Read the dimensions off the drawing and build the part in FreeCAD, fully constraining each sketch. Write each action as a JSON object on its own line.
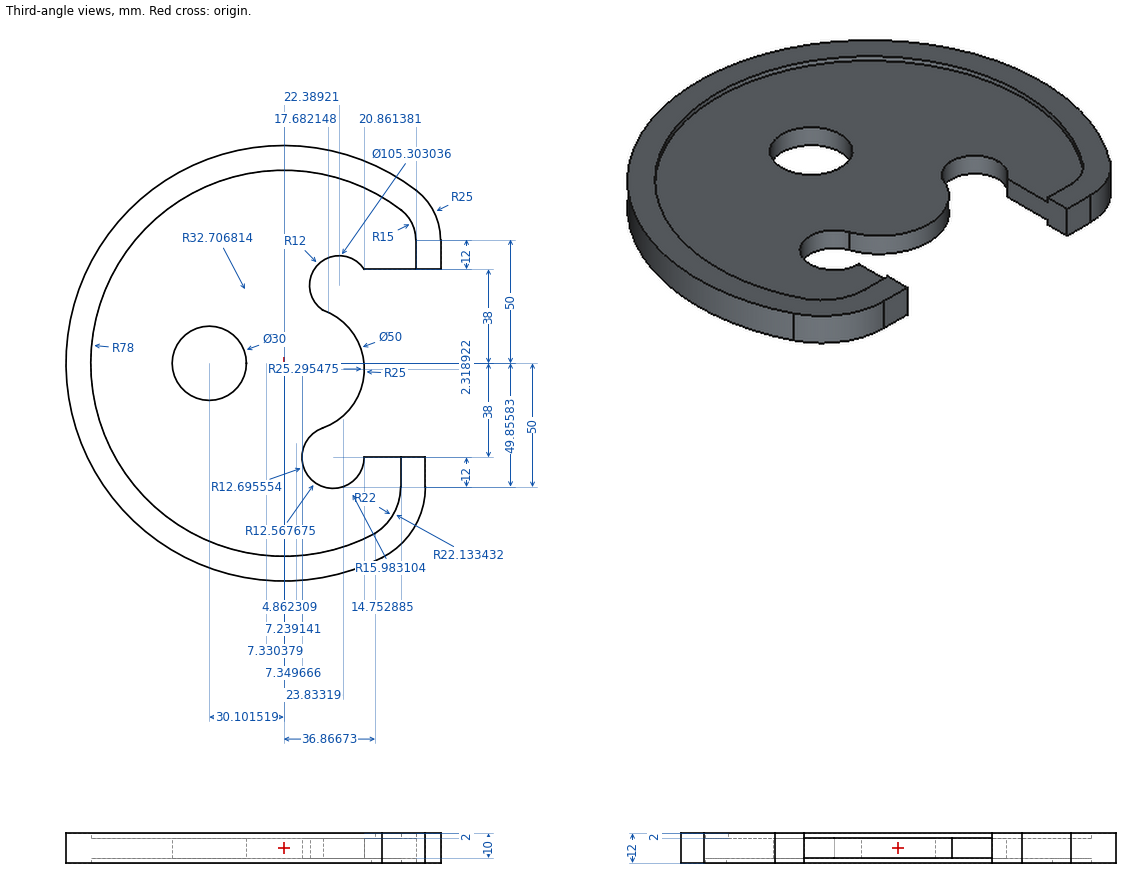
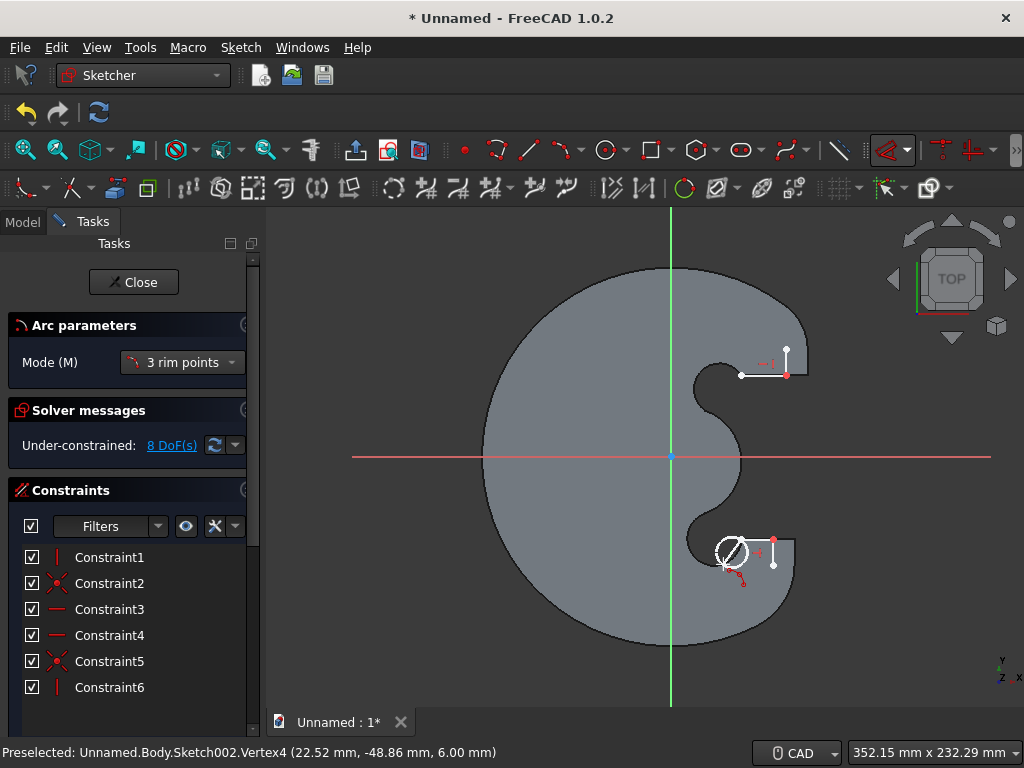
{"action": "scroll", "coordinate": [736, 554], "scroll_direction": "up", "scroll_amount": 6}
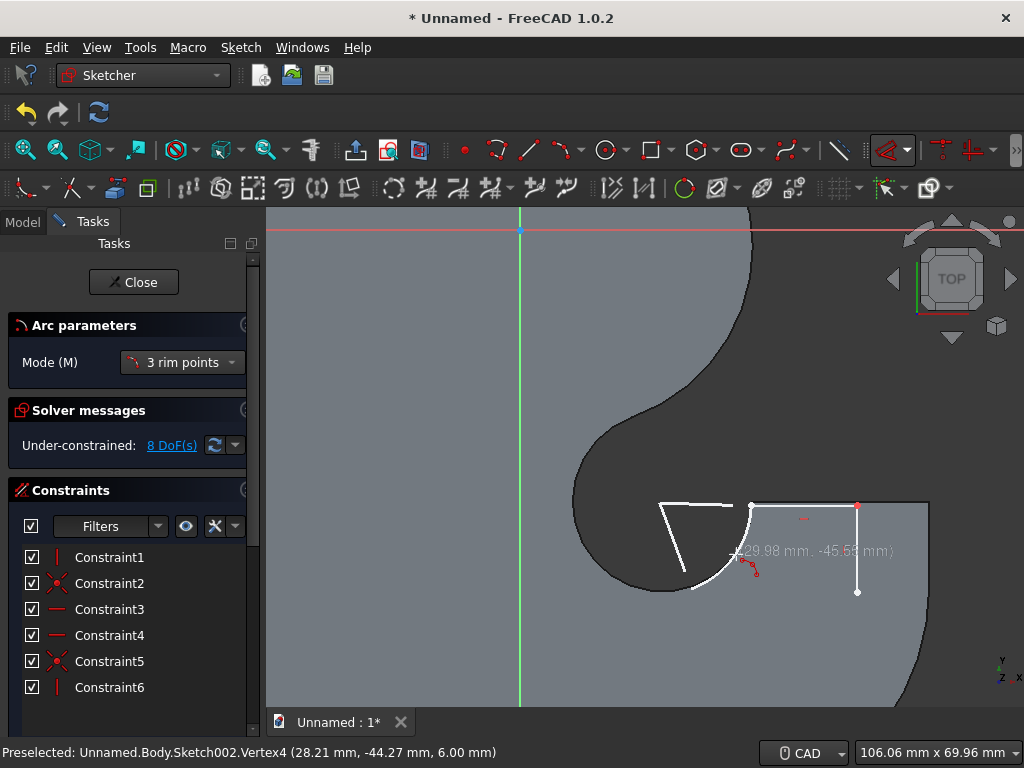
{"action": "left_click", "coordinate": [736, 554]}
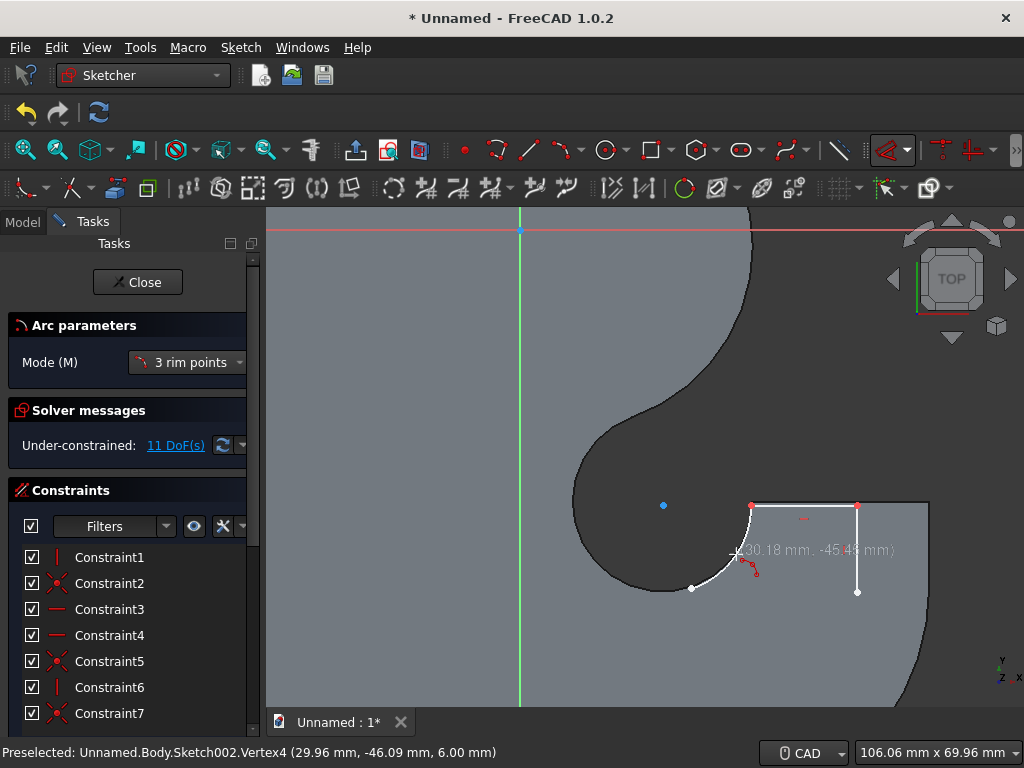
{"action": "left_click", "coordinate": [691, 589]}
{"action": "left_click", "coordinate": [632, 415]}
{"action": "left_click", "coordinate": [577, 531]}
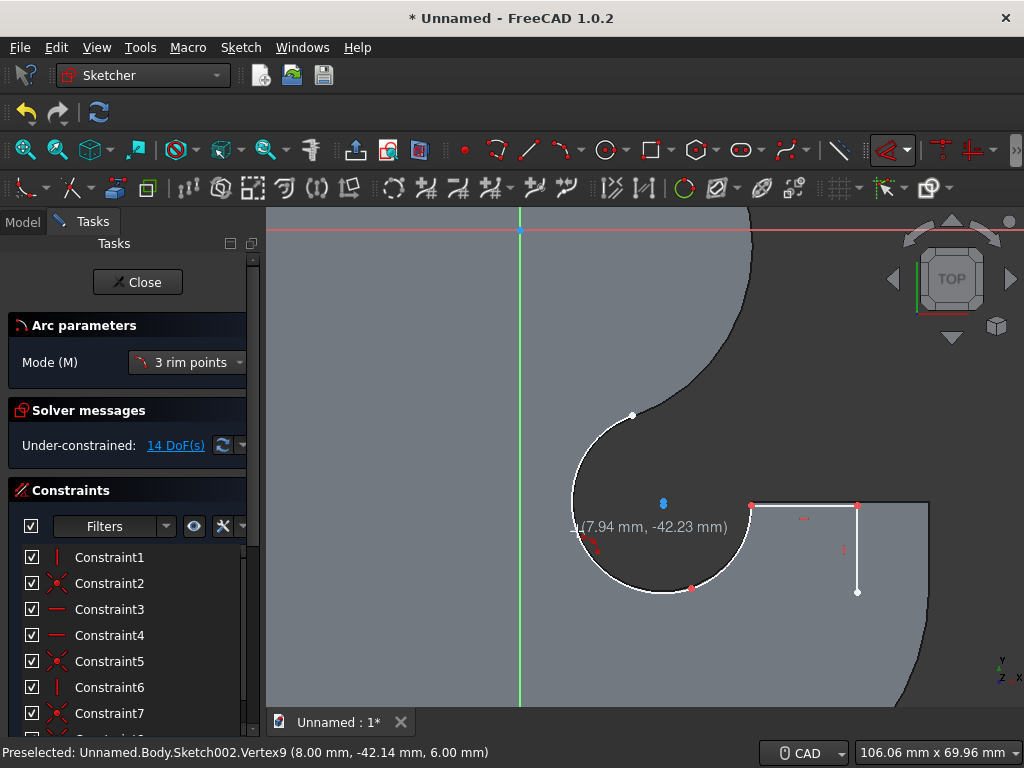
{"action": "left_click", "coordinate": [632, 416]}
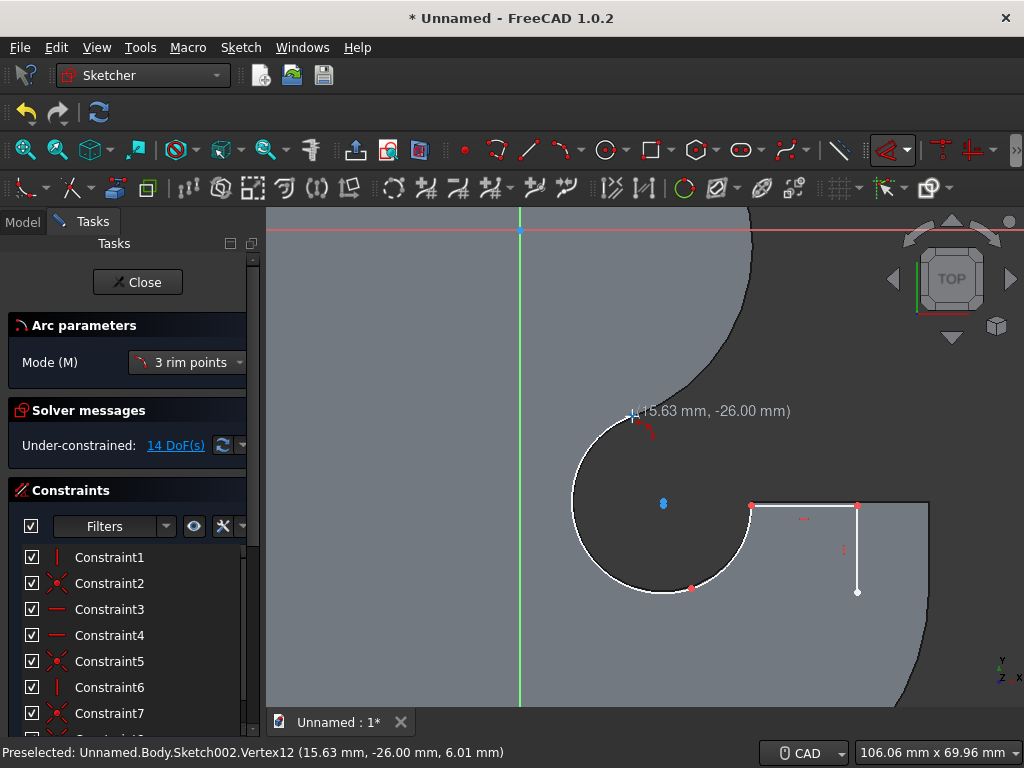
{"action": "scroll", "coordinate": [660, 575], "scroll_direction": "down", "scroll_amount": 5}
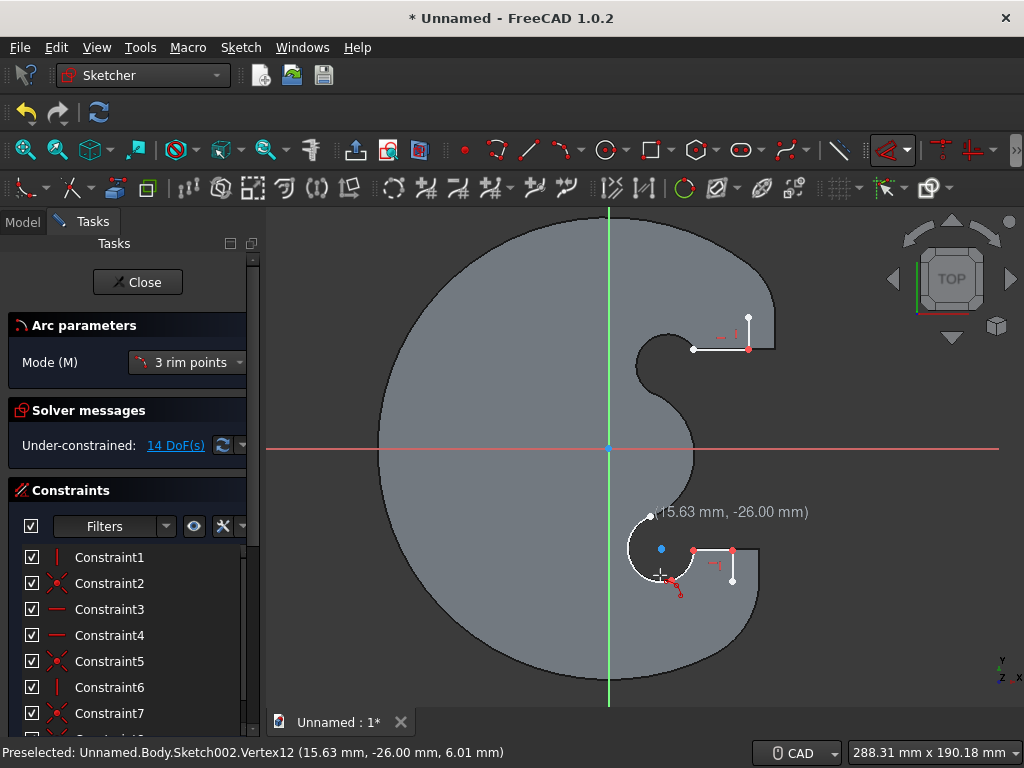
{"action": "left_click", "coordinate": [655, 395]}
{"action": "left_click", "coordinate": [691, 473]}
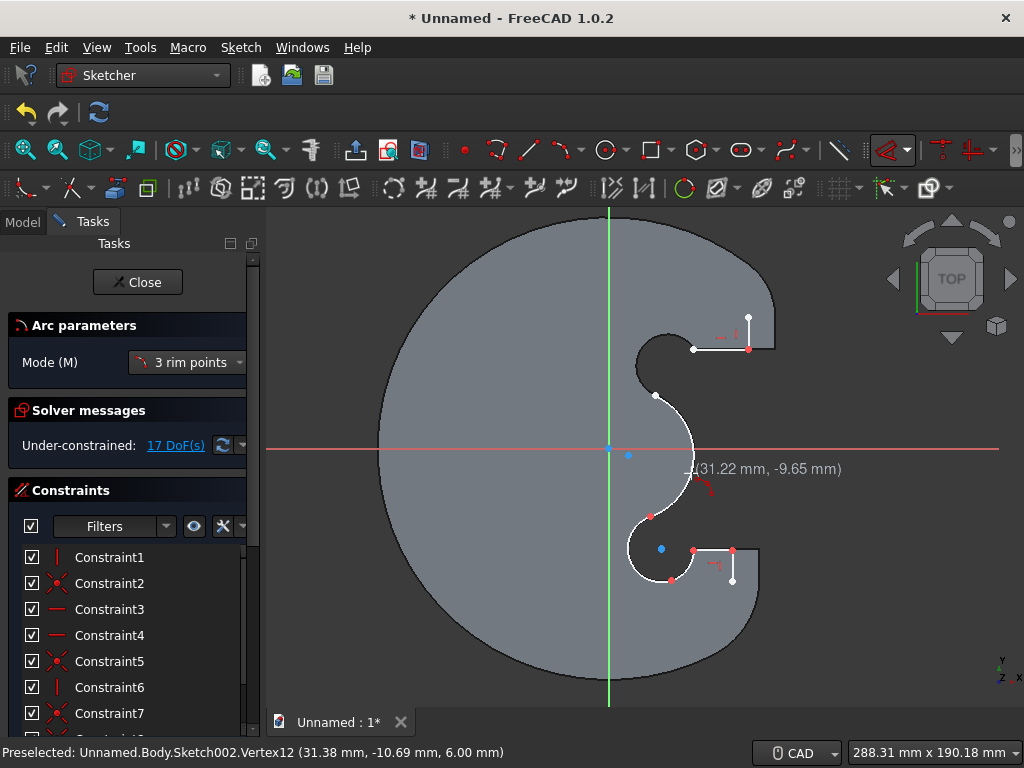
{"action": "left_click", "coordinate": [655, 396]}
{"action": "left_click", "coordinate": [694, 350]}
{"action": "left_click", "coordinate": [644, 346]}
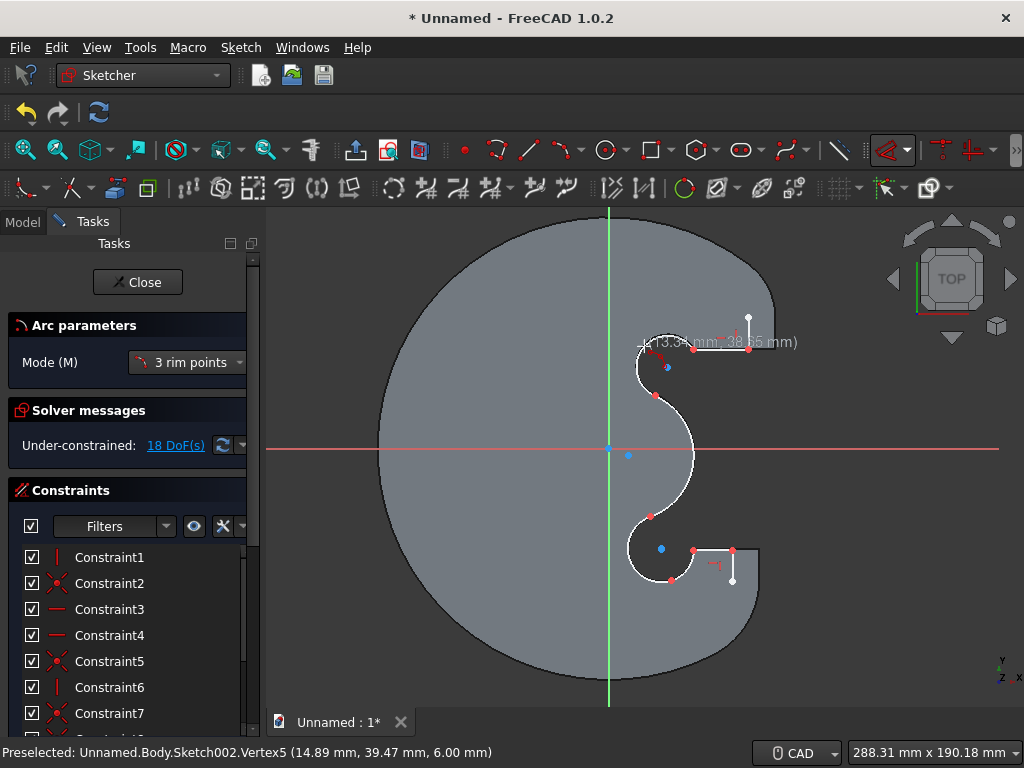
{"action": "left_click", "coordinate": [749, 318]}
{"action": "left_click", "coordinate": [734, 286]}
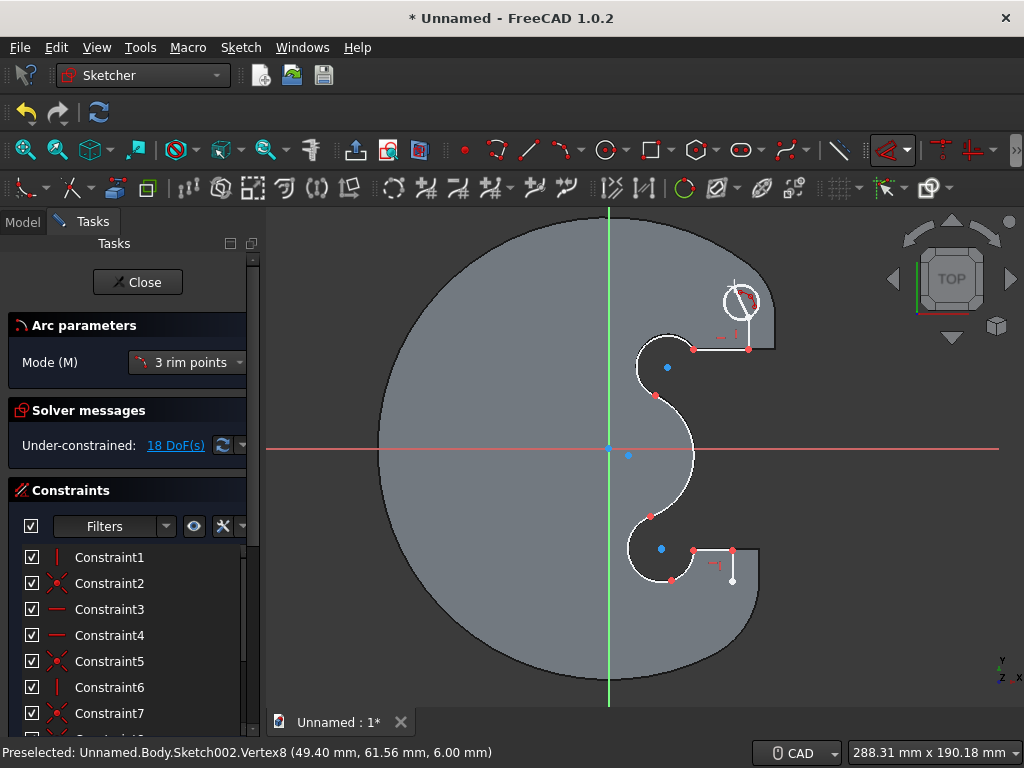
{"action": "scroll", "coordinate": [745, 300], "scroll_direction": "up", "scroll_amount": 7}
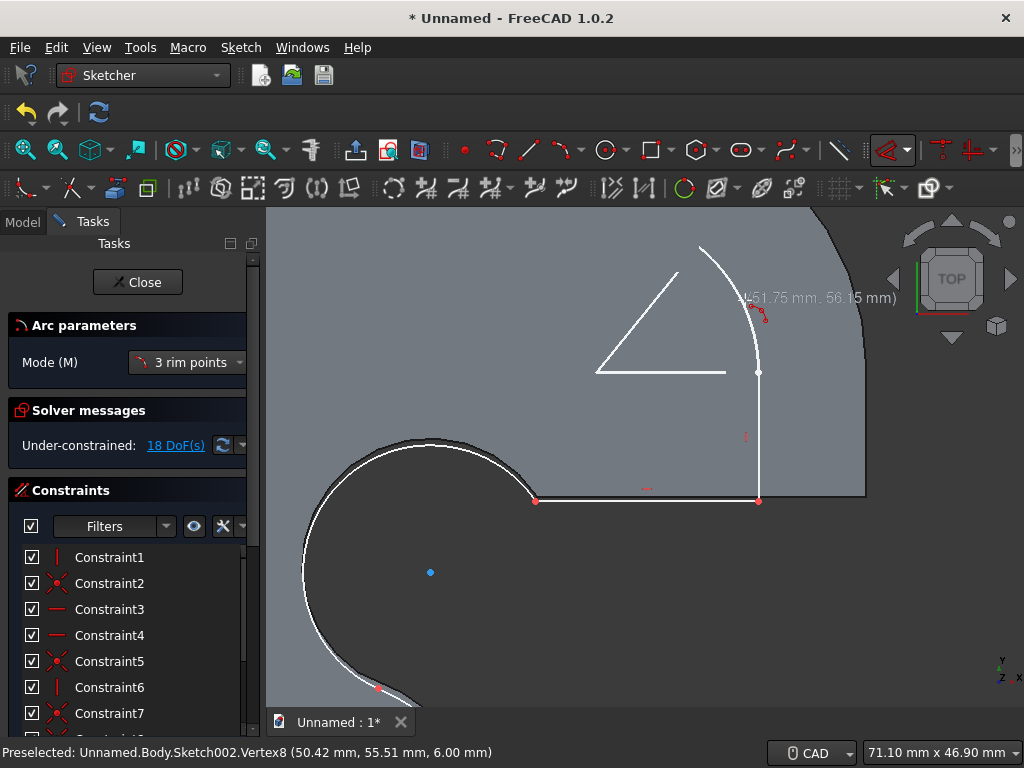
{"action": "left_click", "coordinate": [743, 298]}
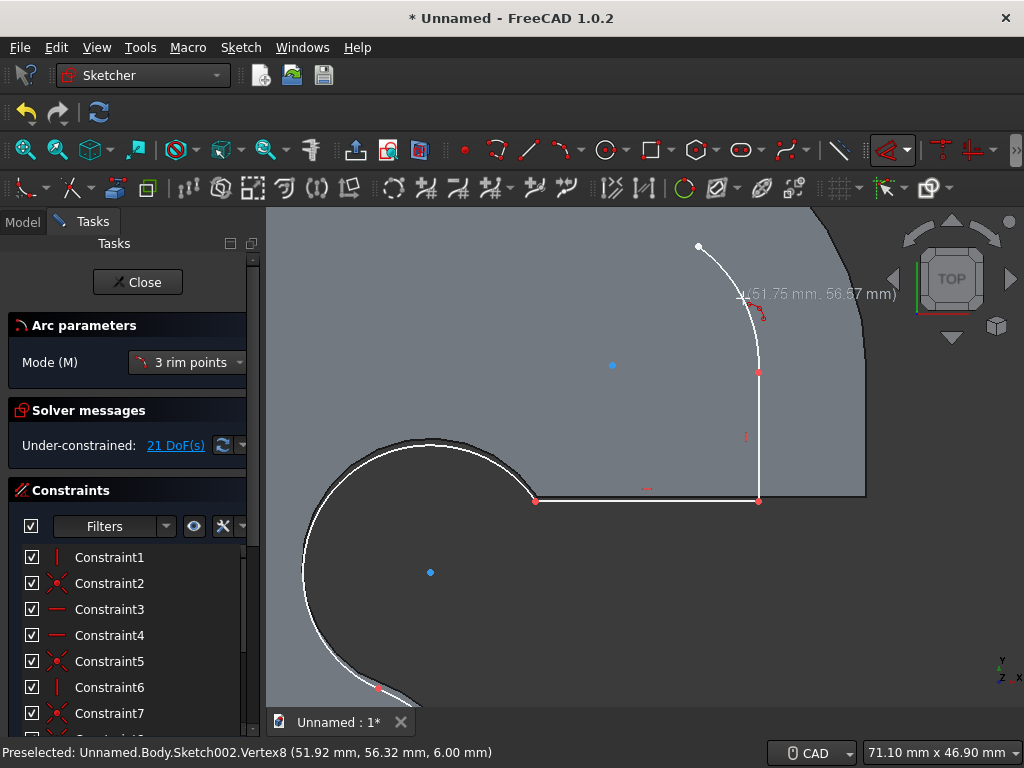
{"action": "scroll", "coordinate": [745, 299], "scroll_direction": "down", "scroll_amount": 7}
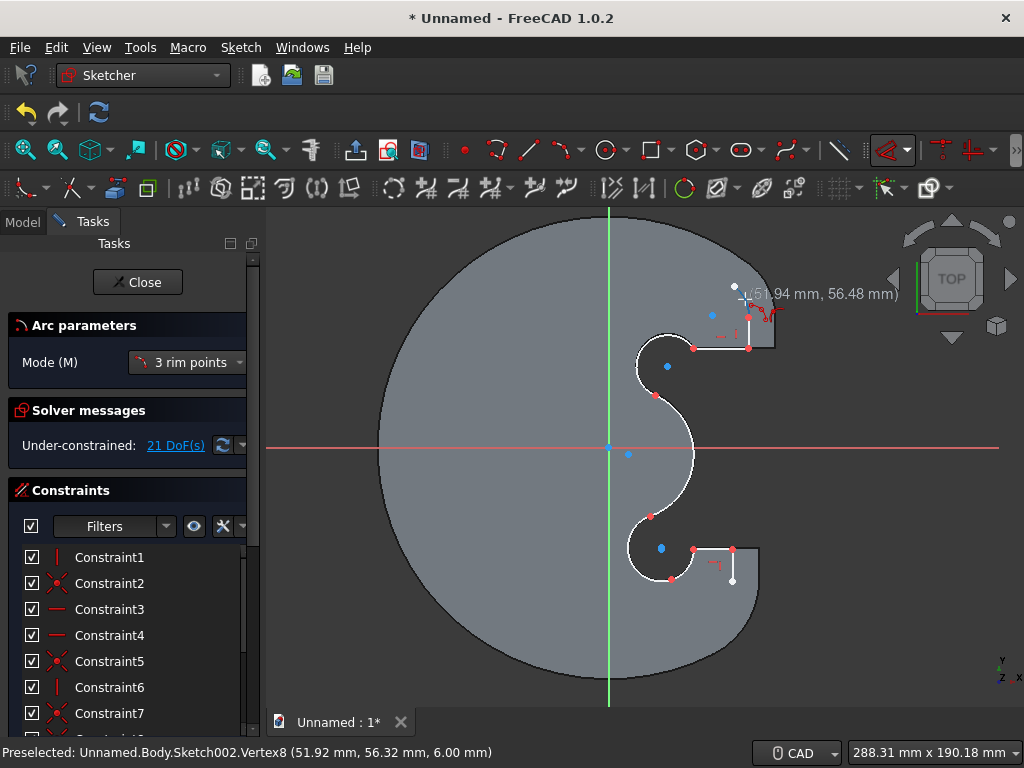
{"action": "left_click", "coordinate": [734, 286]}
{"action": "left_click", "coordinate": [706, 629]}
{"action": "left_click", "coordinate": [430, 348]}